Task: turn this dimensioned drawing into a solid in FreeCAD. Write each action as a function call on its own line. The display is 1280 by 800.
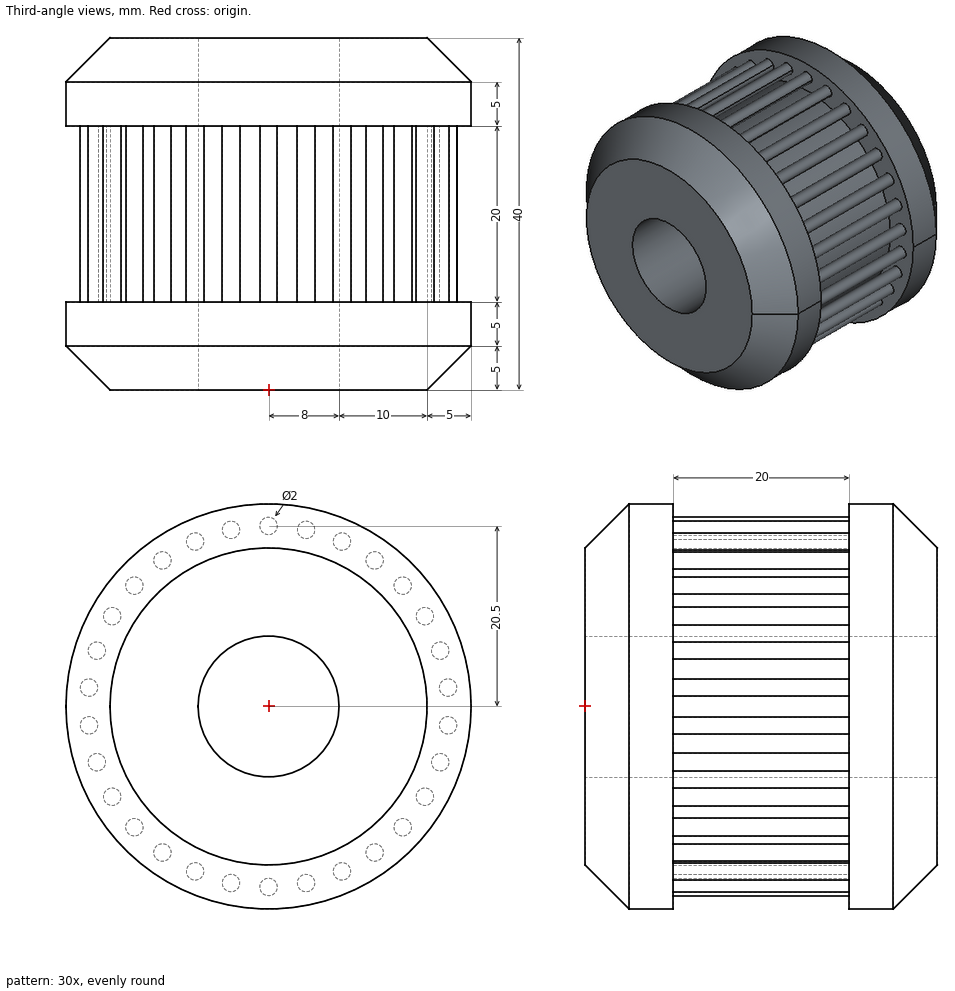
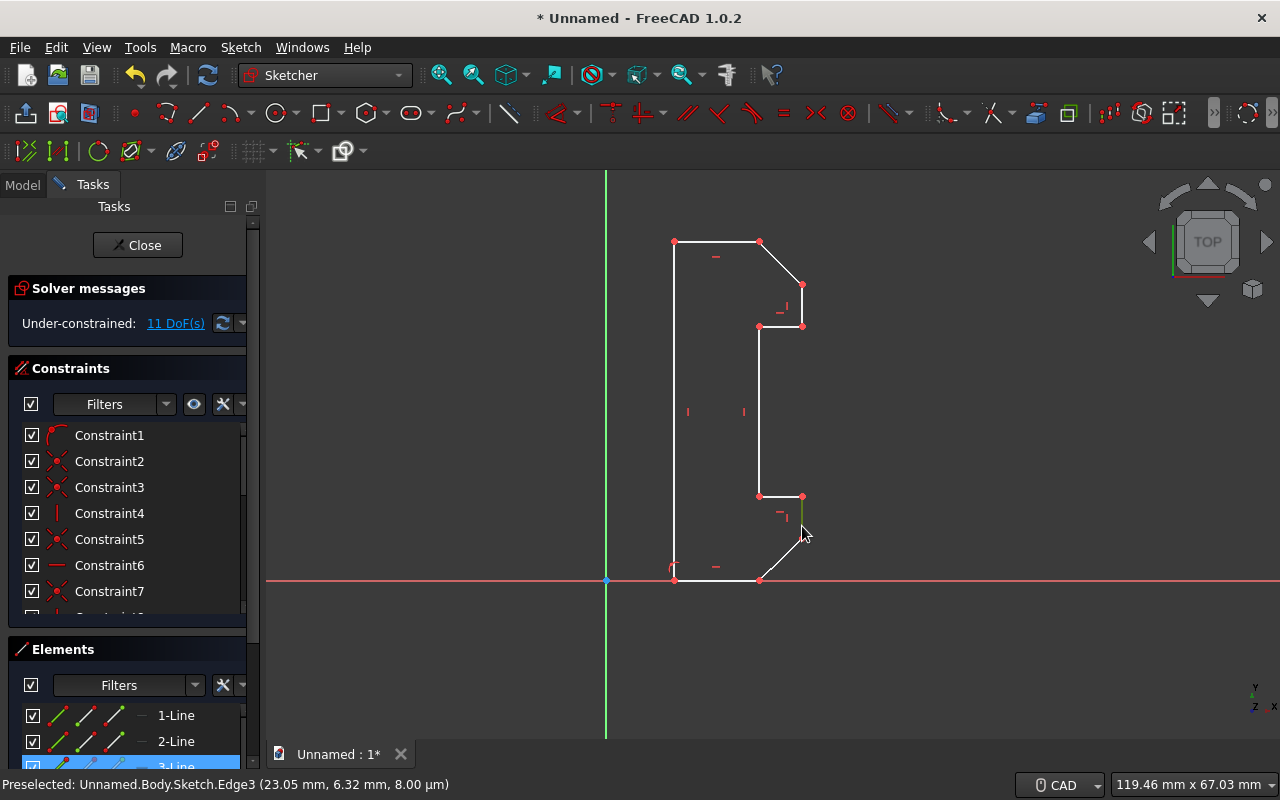
key(i)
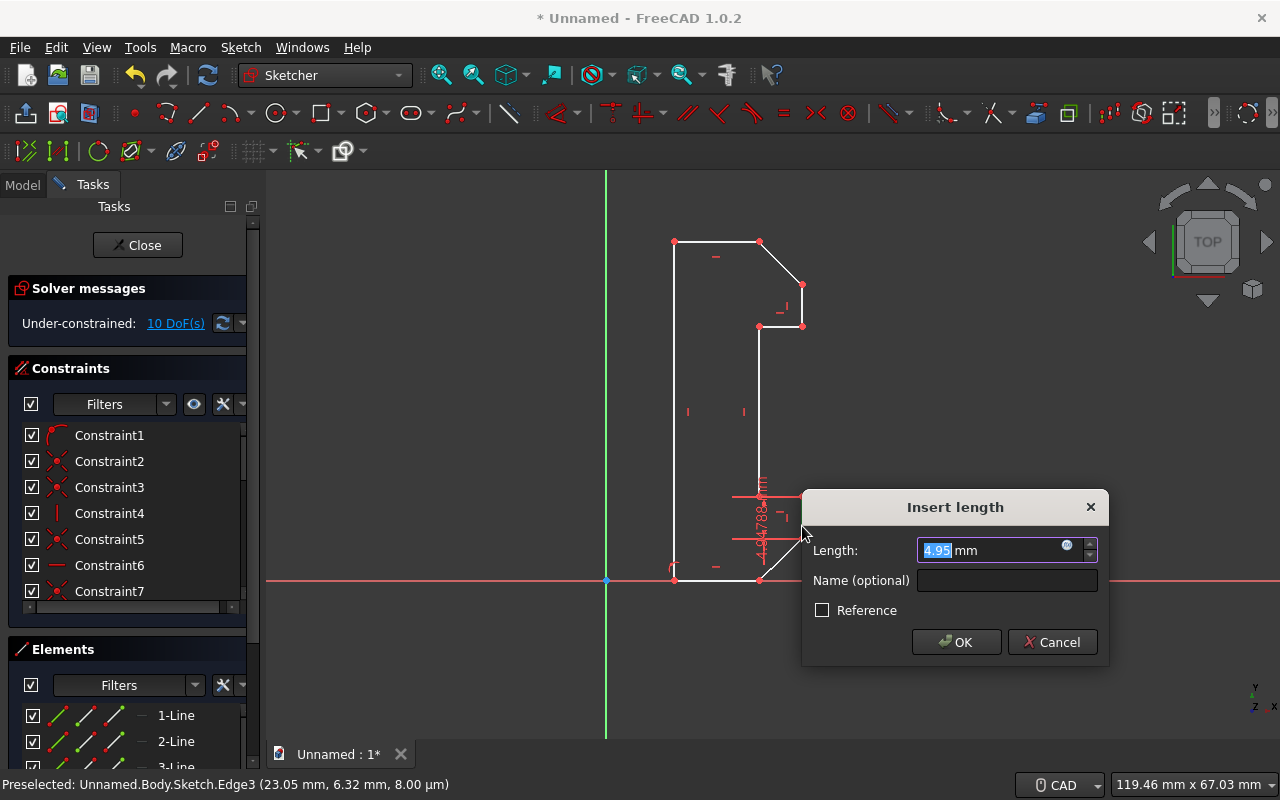
text(5)
key(Return)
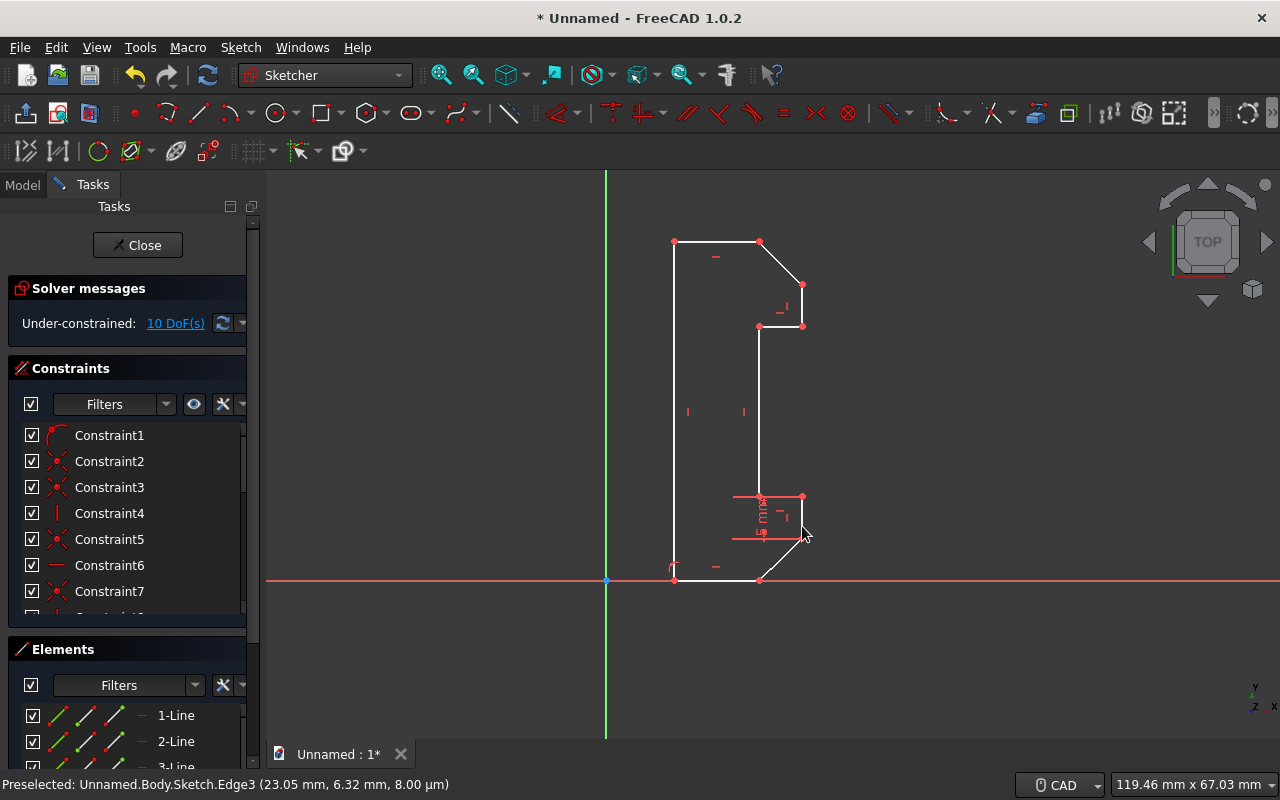
click(789, 497)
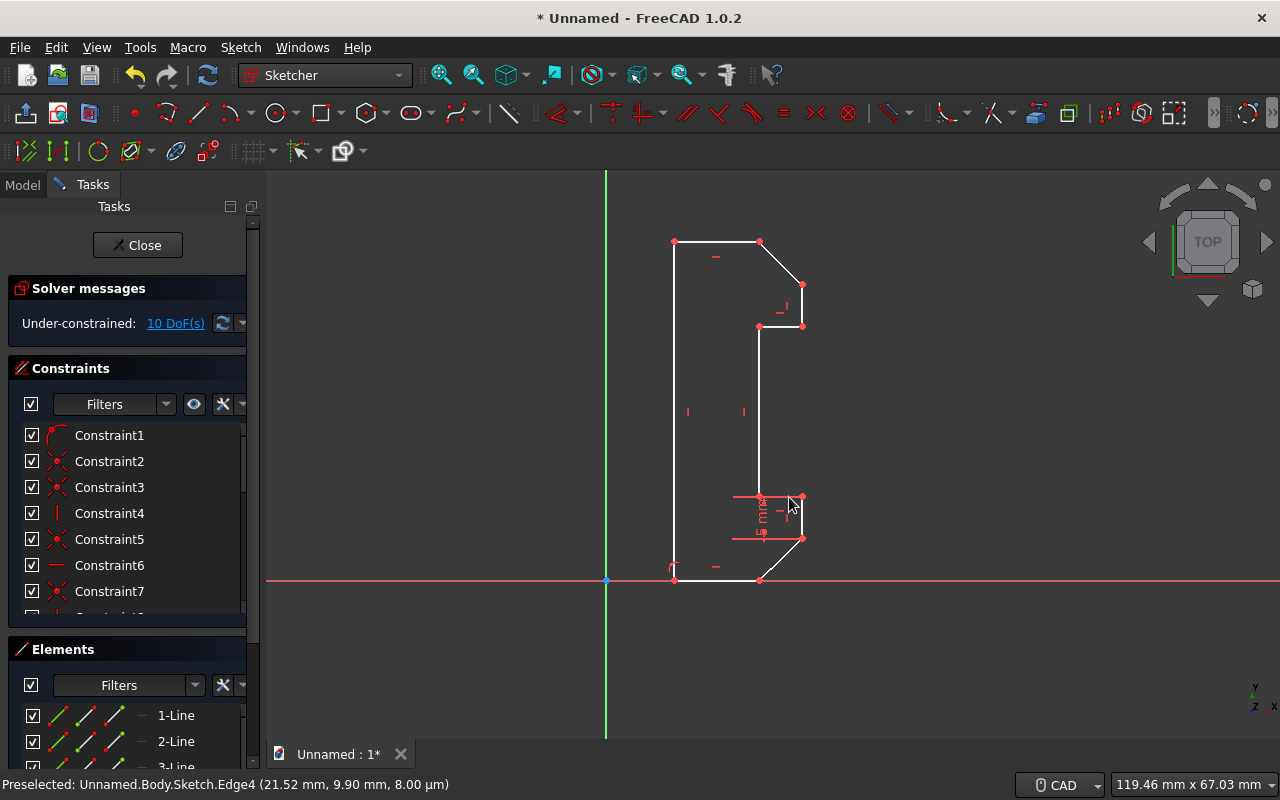
key(l)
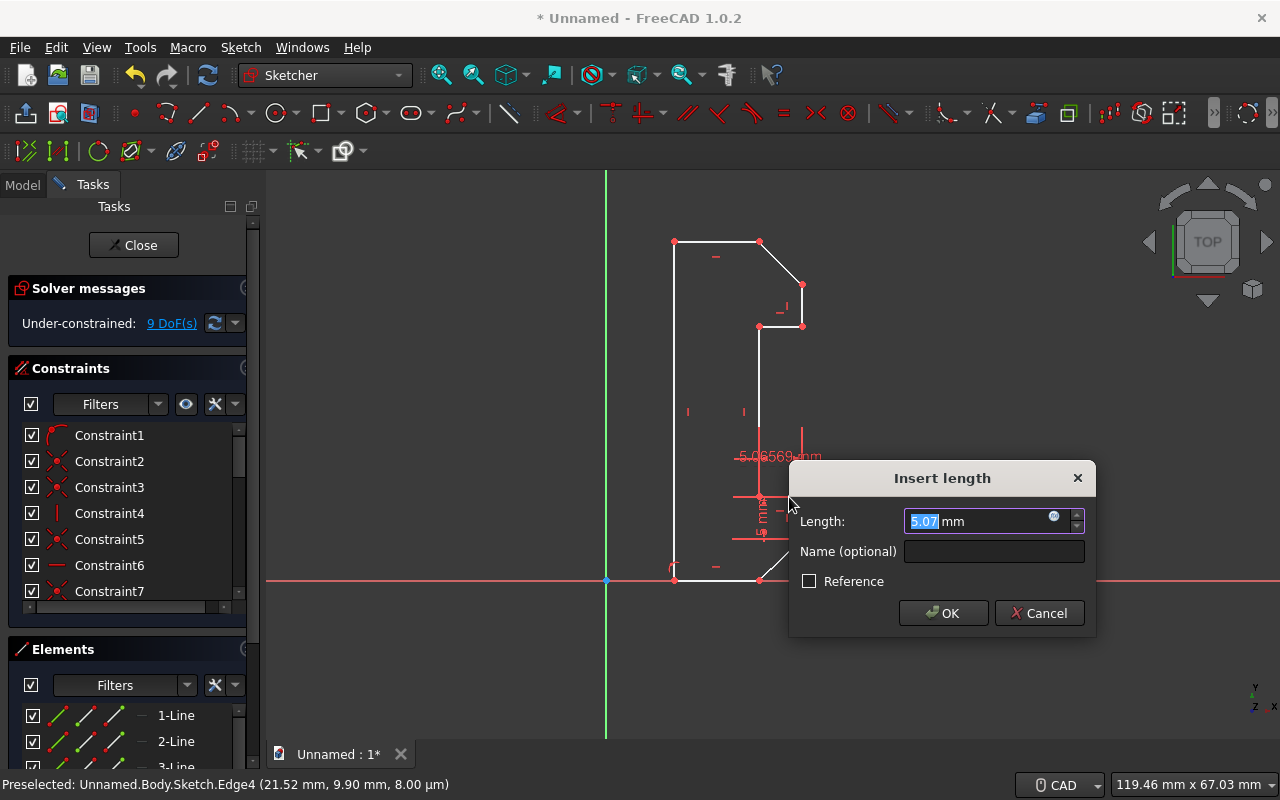
text(5)
key(Return)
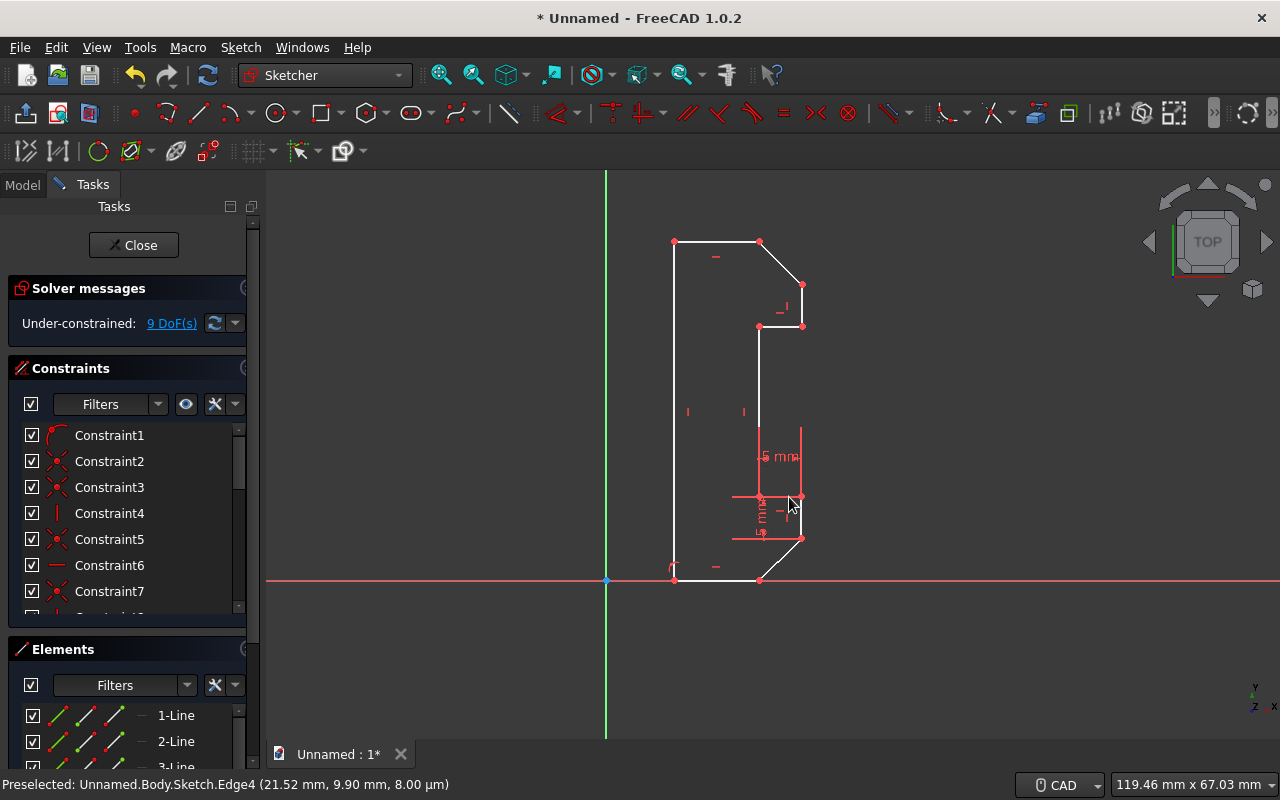
click(772, 327)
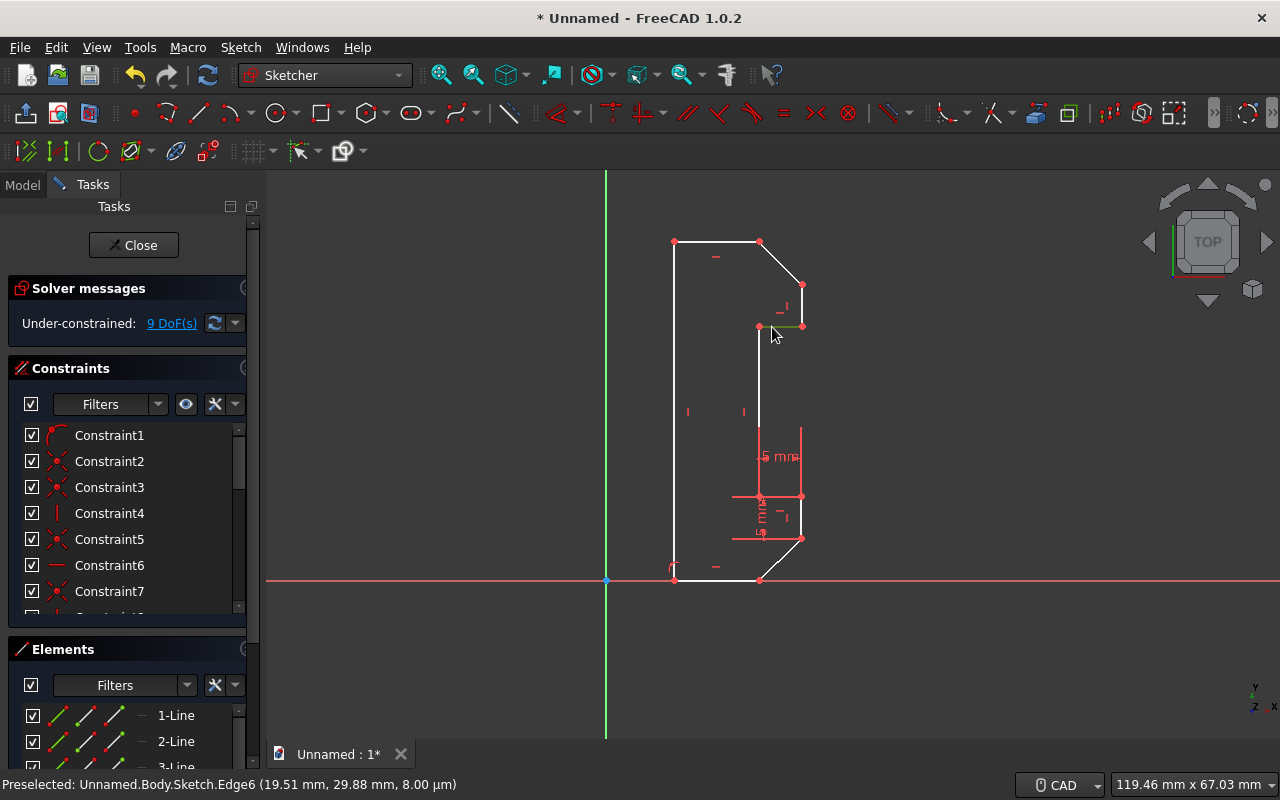
key(l)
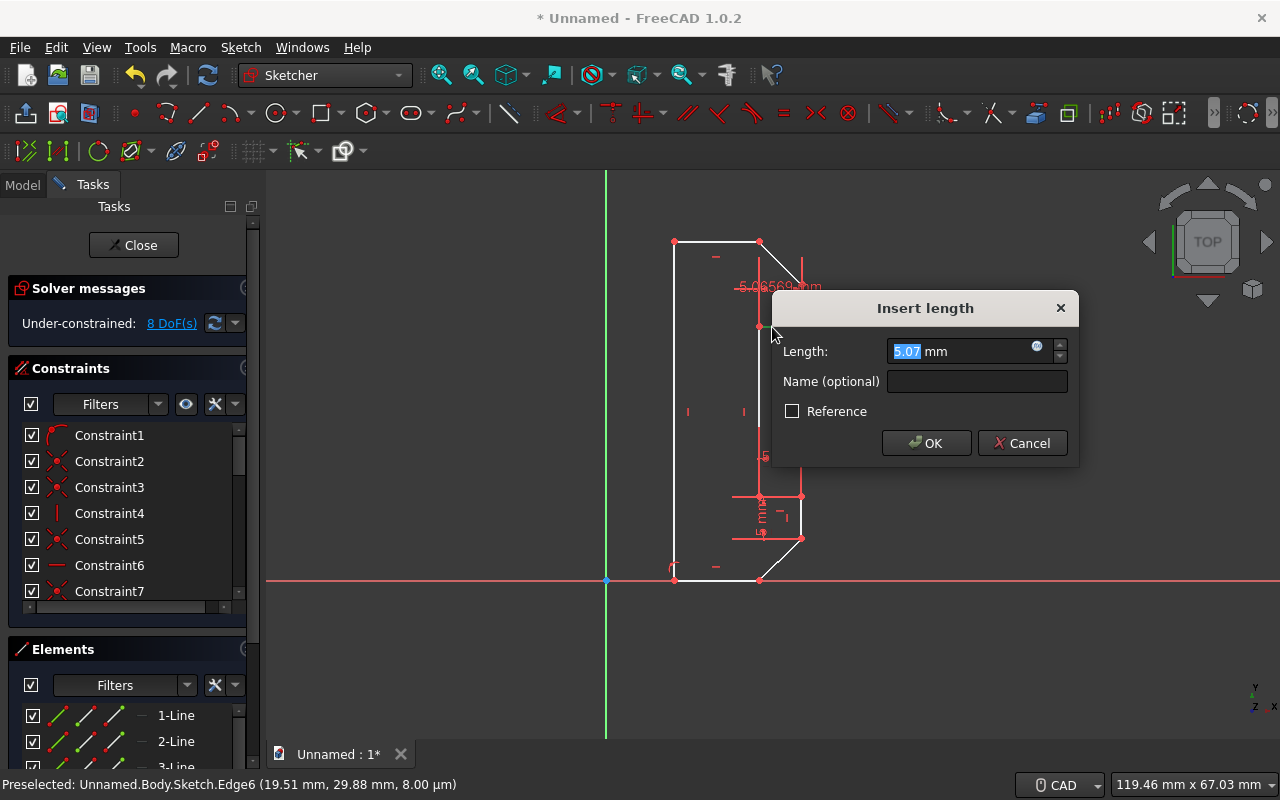
text(5)
key(Return)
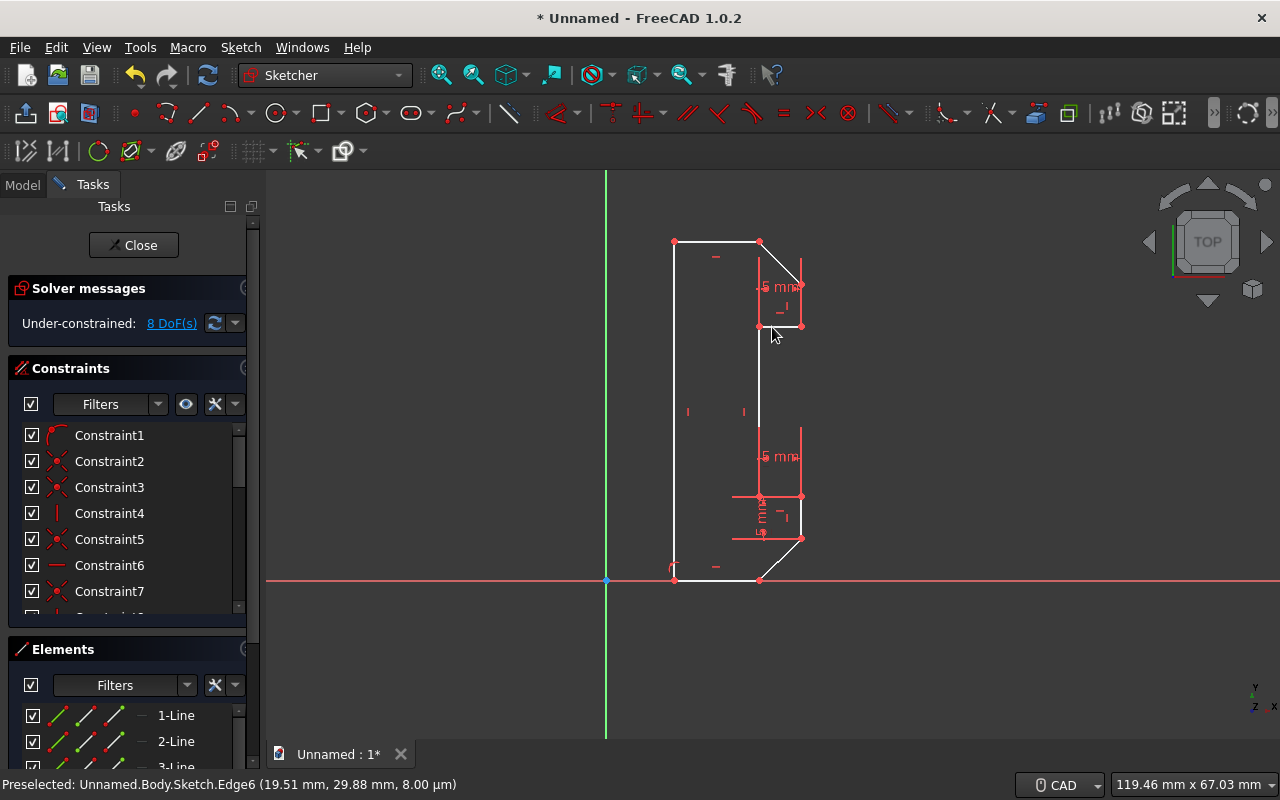
click(801, 314)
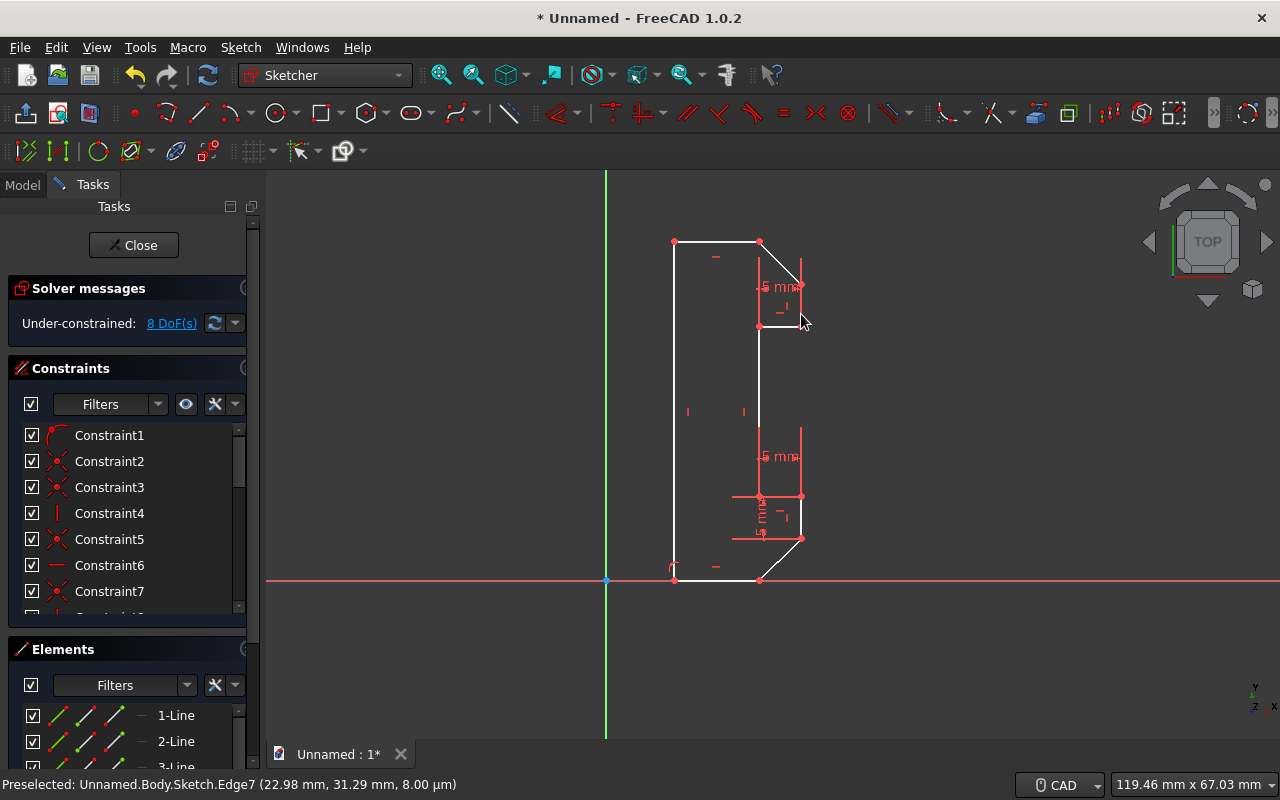
click(580, 114)